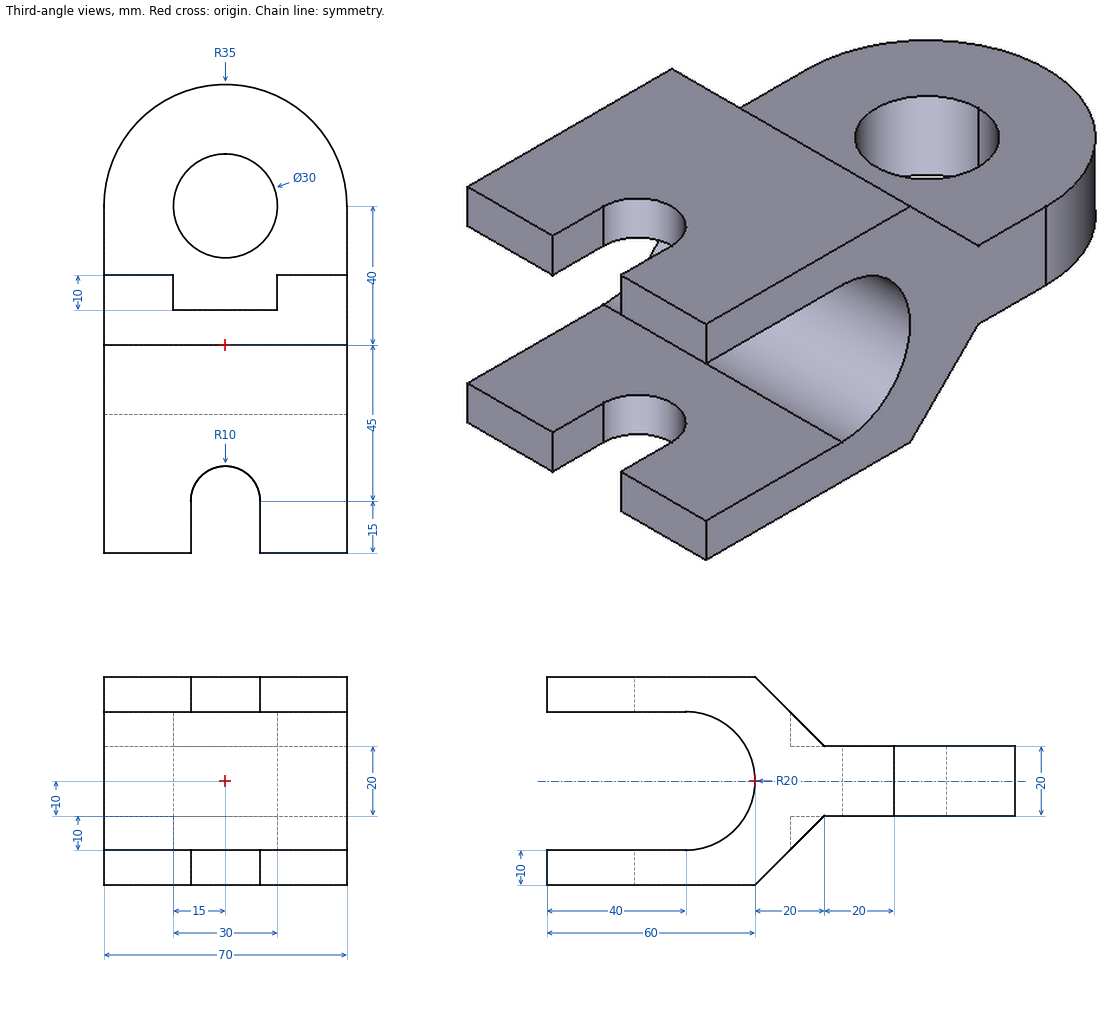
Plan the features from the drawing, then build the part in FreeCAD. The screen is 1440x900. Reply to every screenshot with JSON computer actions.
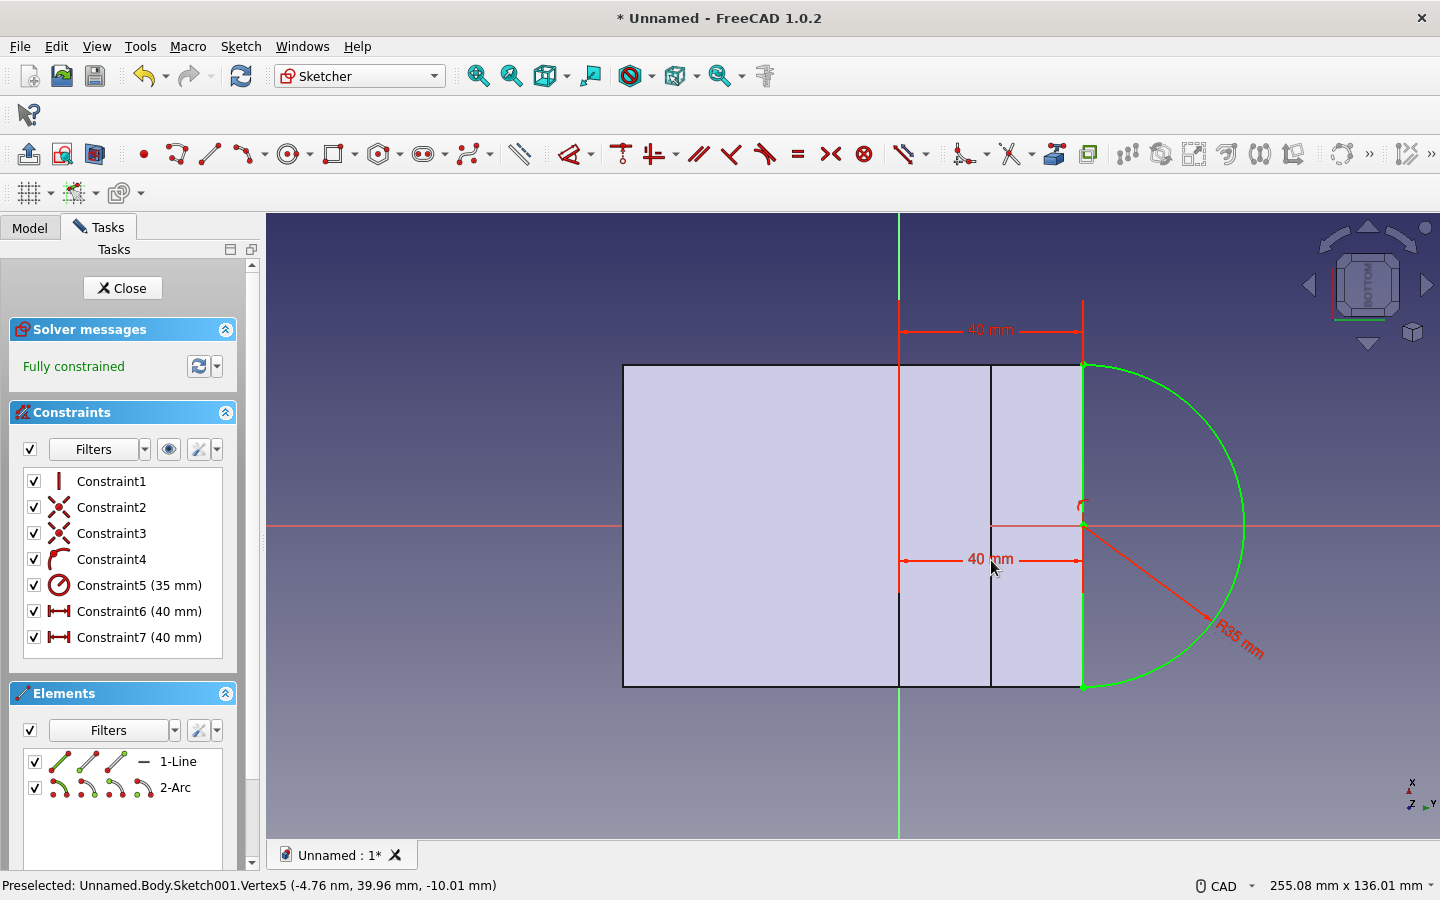
{"action": "left_click", "coordinate": [123, 288]}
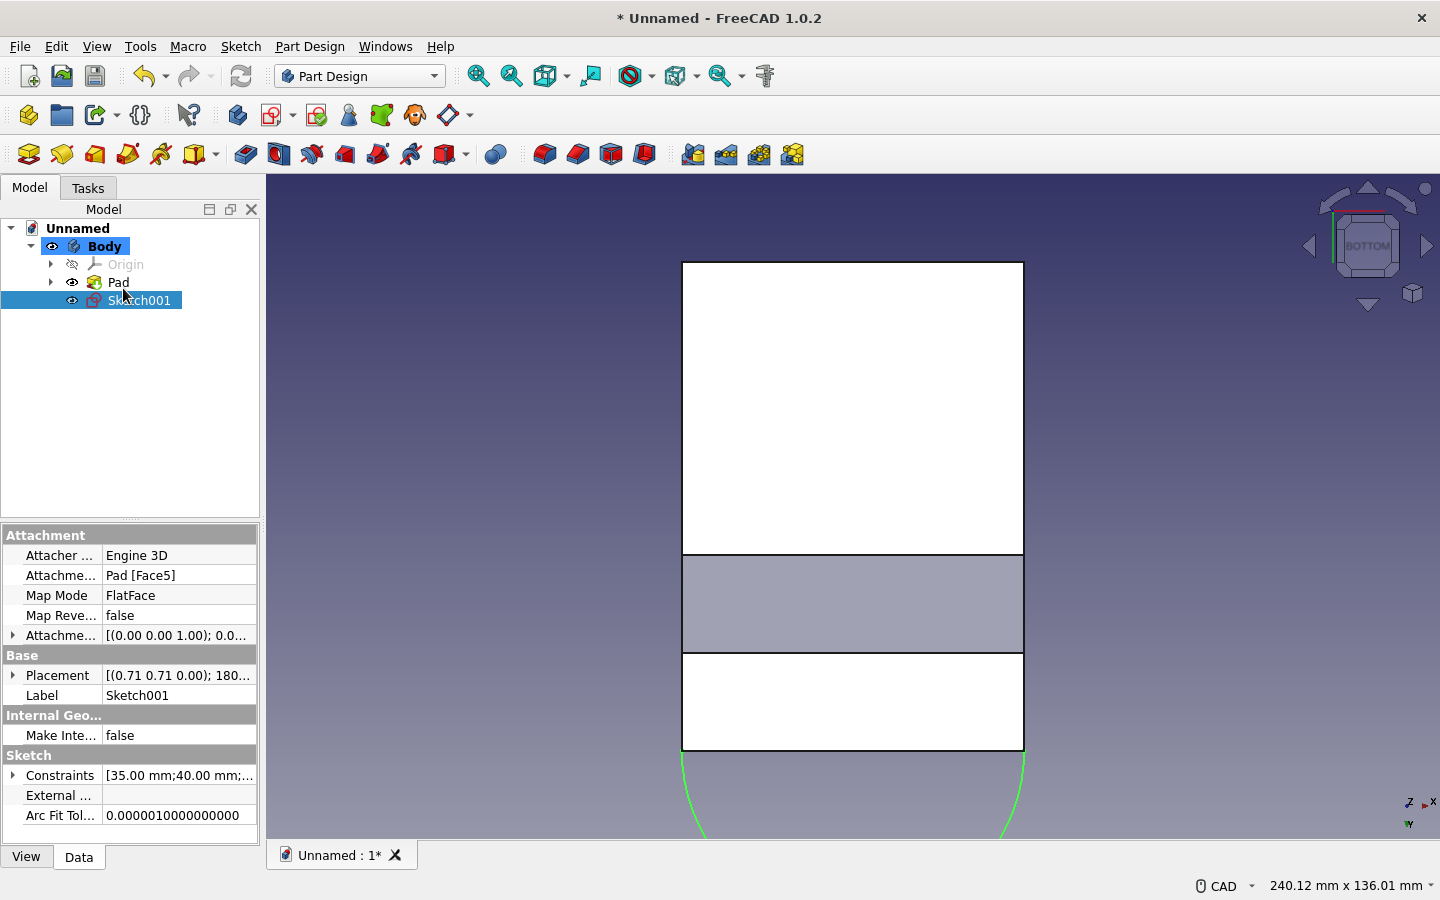
{"action": "left_click", "coordinate": [29, 154]}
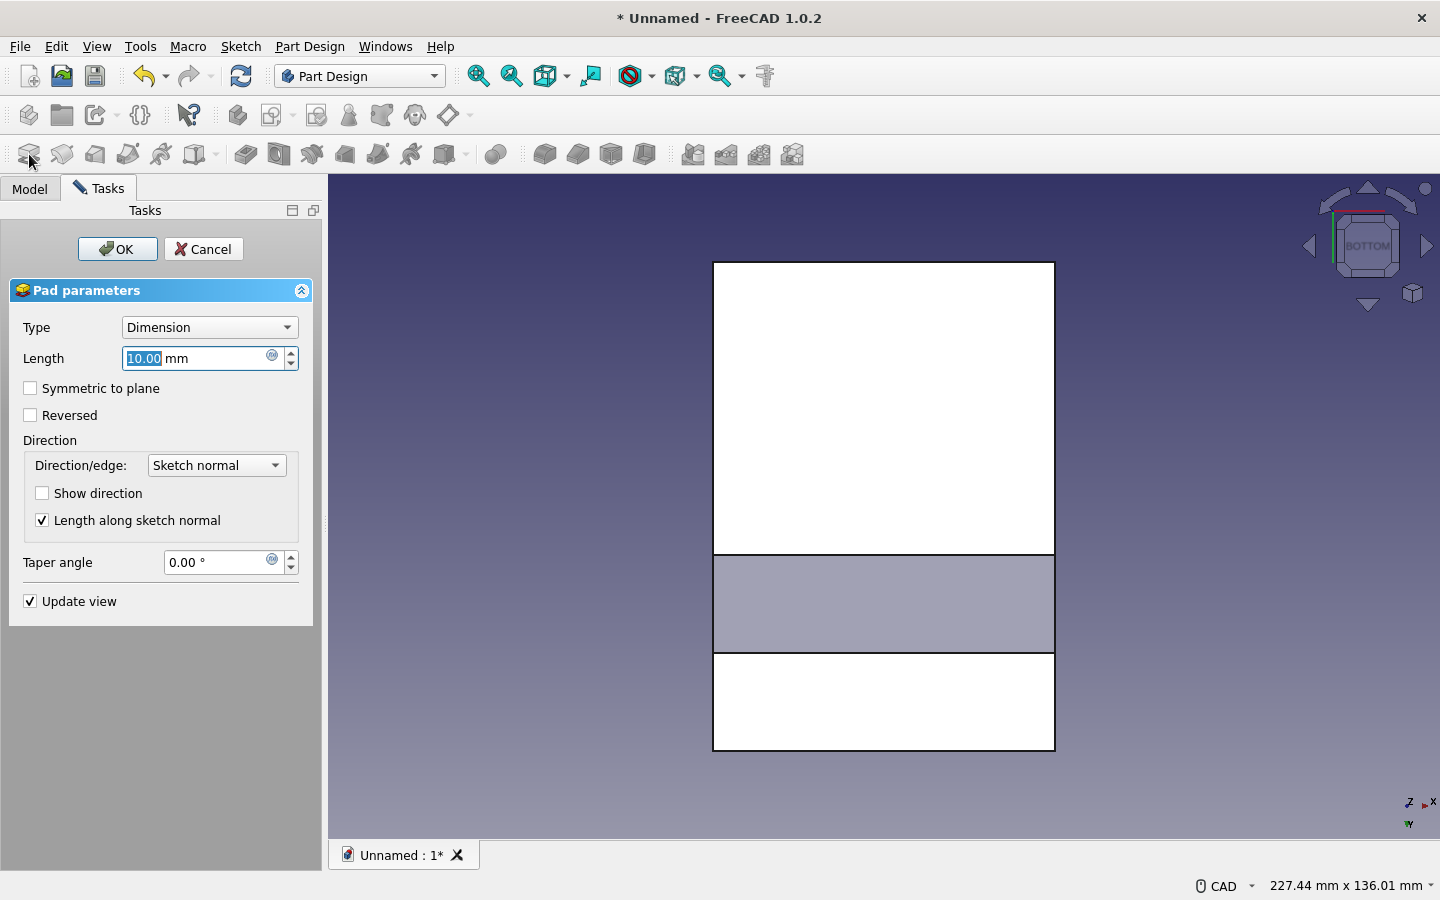
{"action": "type", "text": "20"}
{"action": "key", "text": "Tab"}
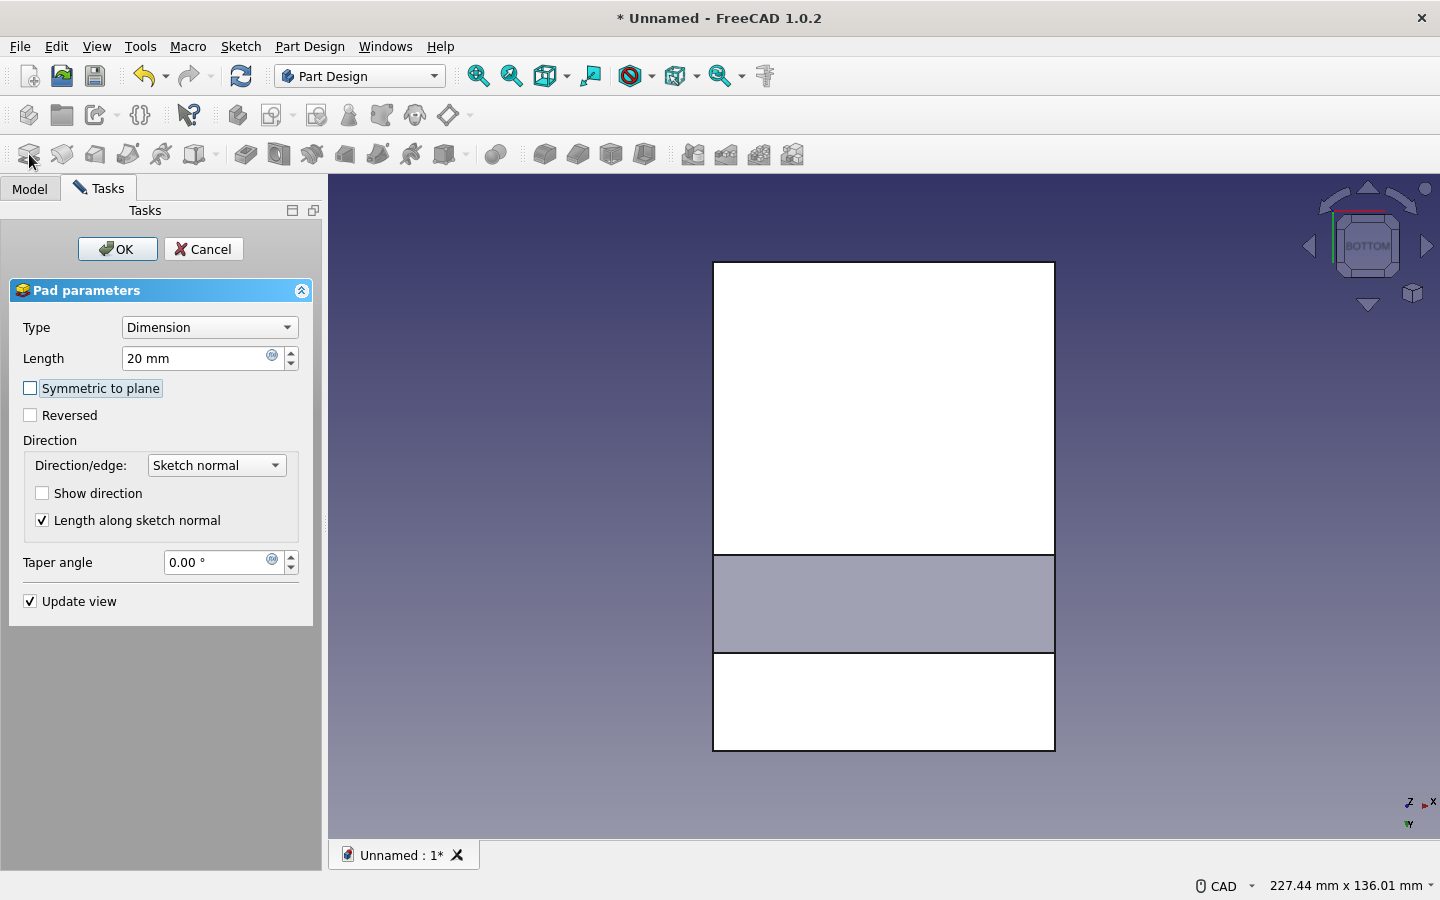
{"action": "left_click", "coordinate": [31, 415]}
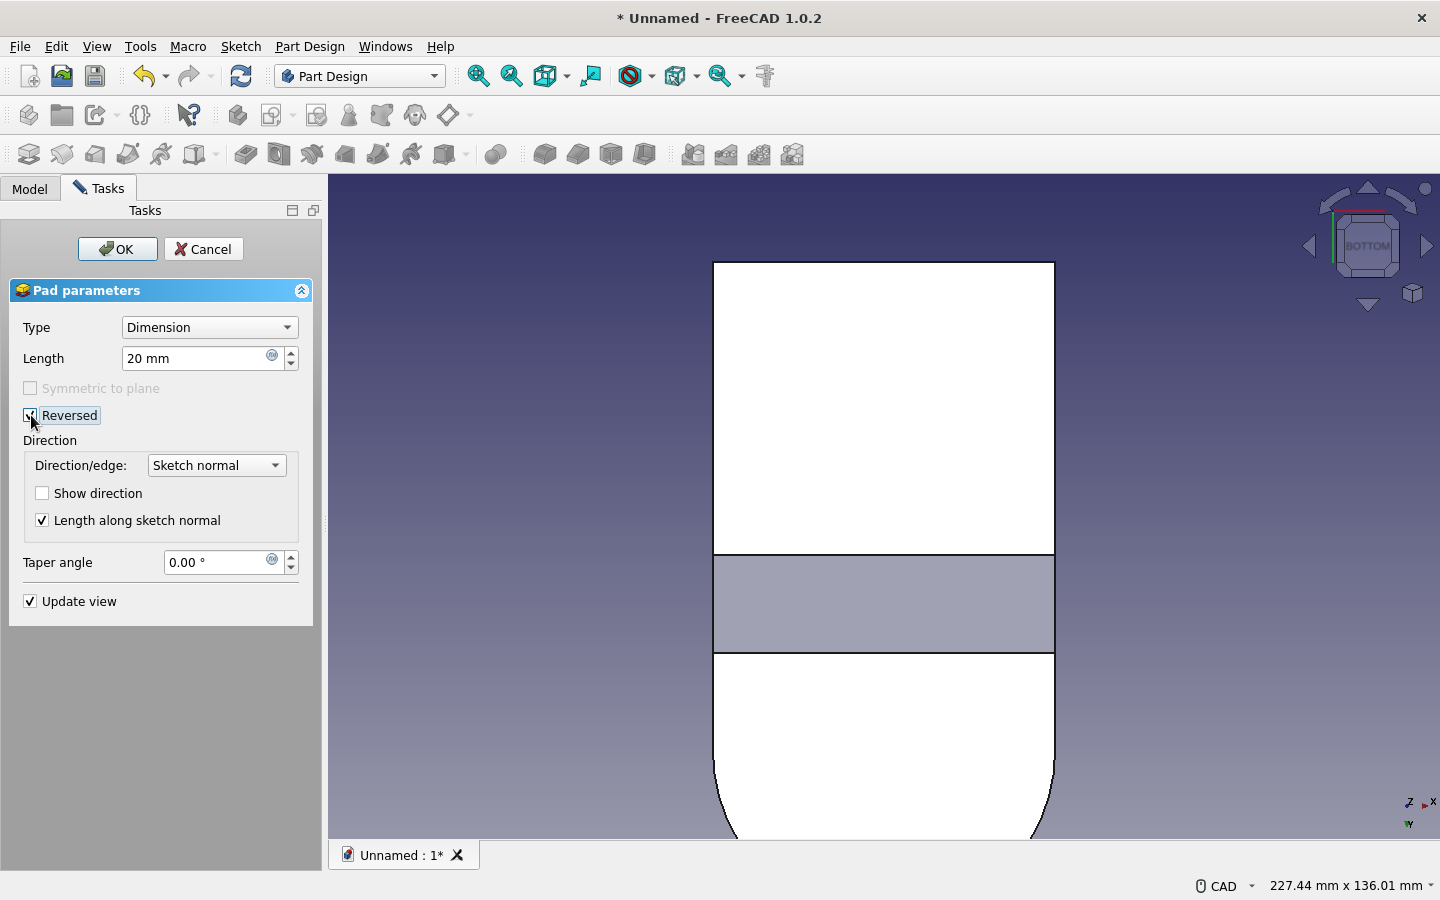
{"action": "left_click", "coordinate": [118, 249]}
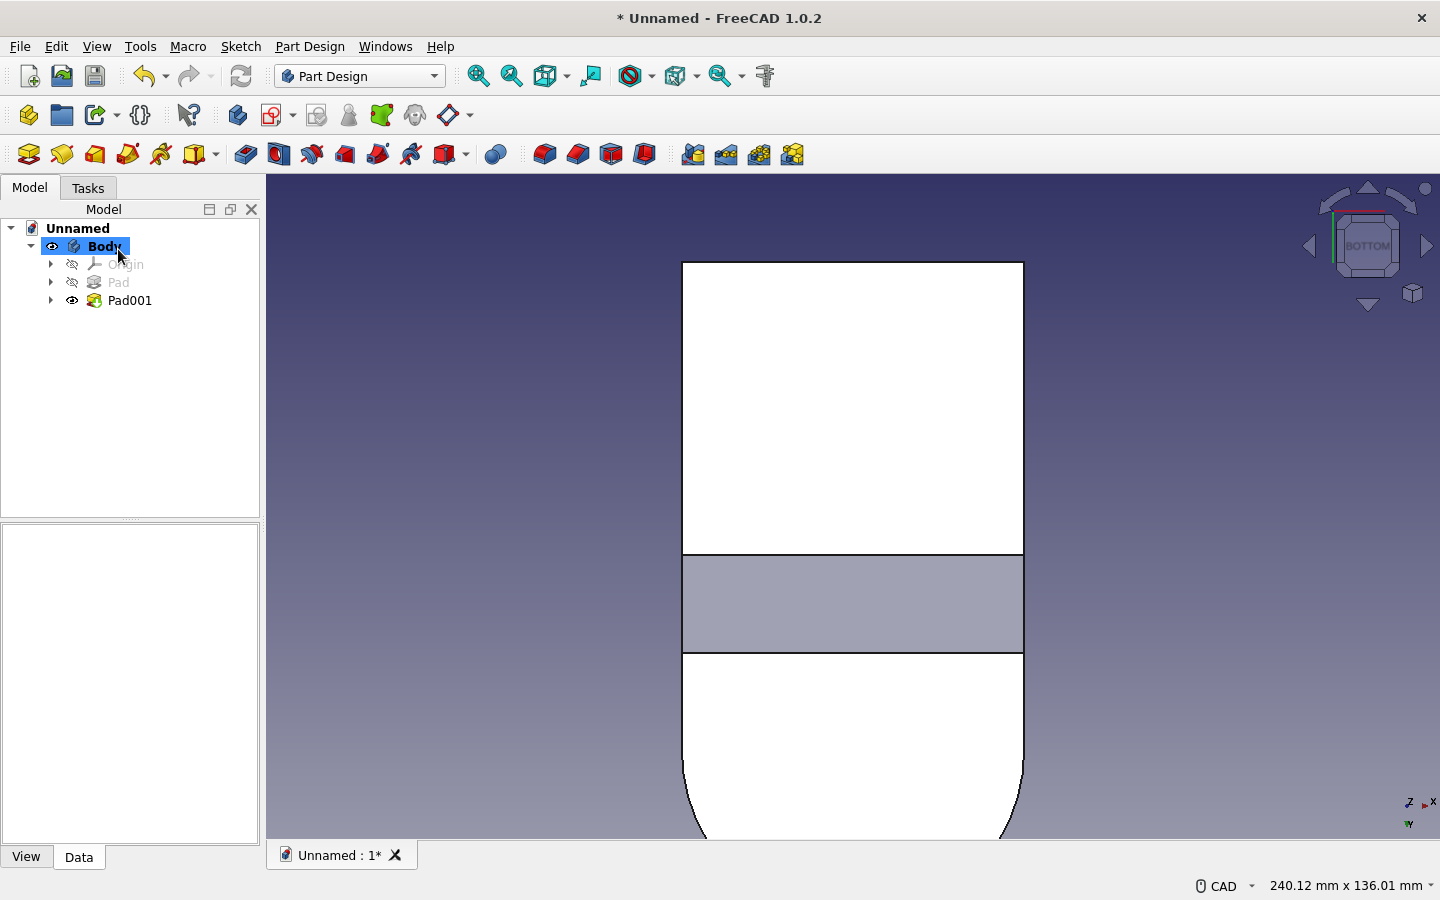
{"action": "key", "text": "v f"}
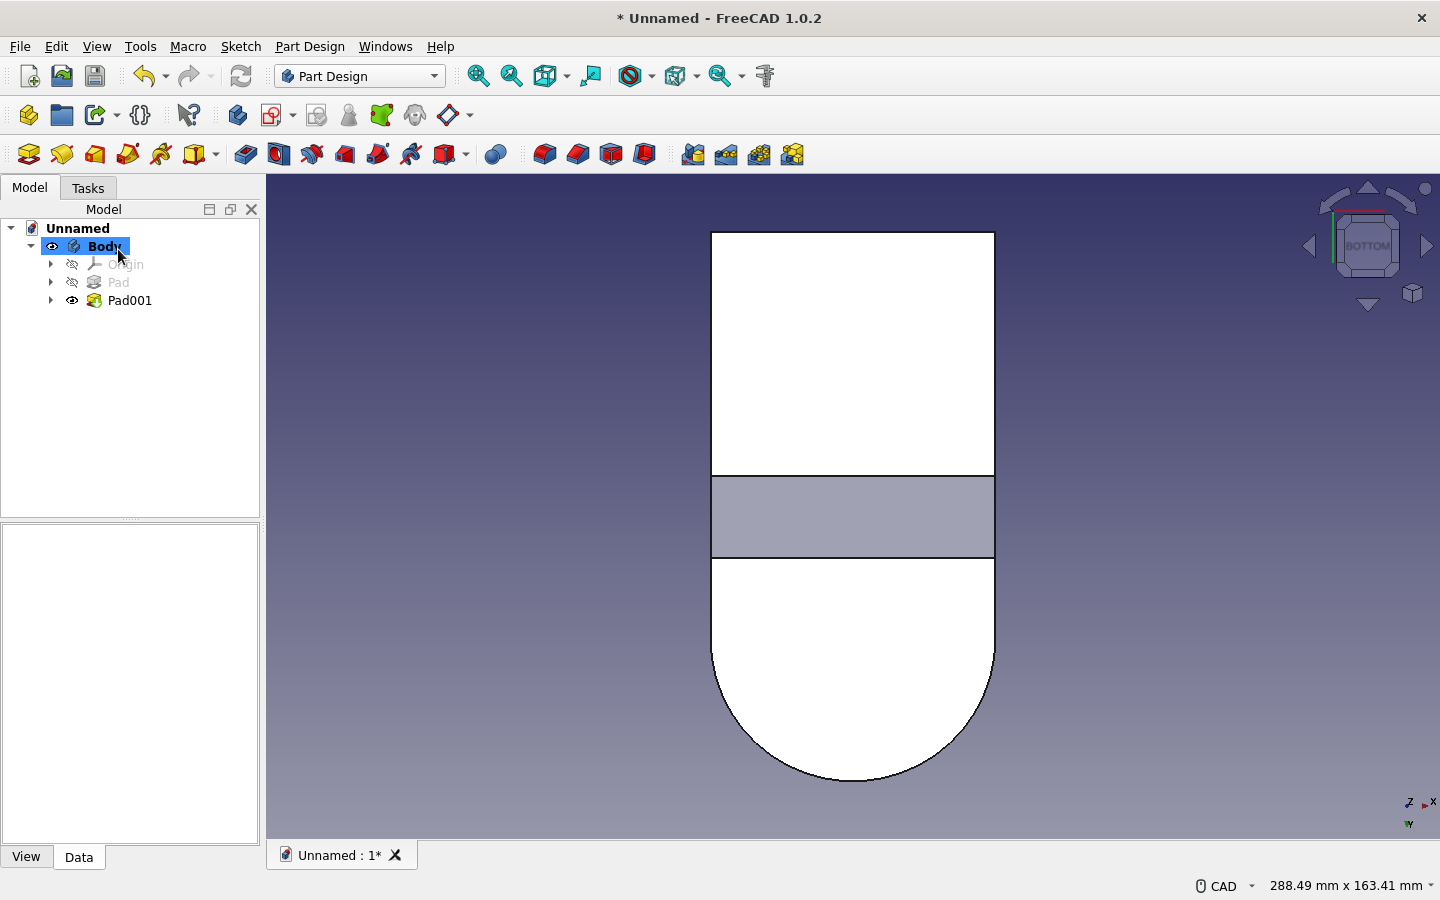
{"action": "left_click", "coordinate": [853, 668]}